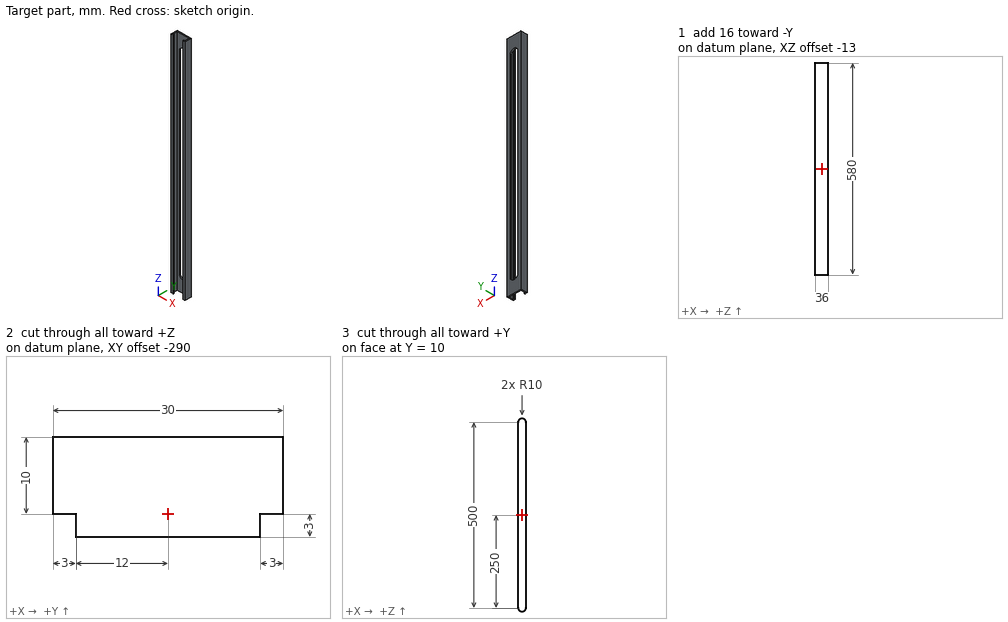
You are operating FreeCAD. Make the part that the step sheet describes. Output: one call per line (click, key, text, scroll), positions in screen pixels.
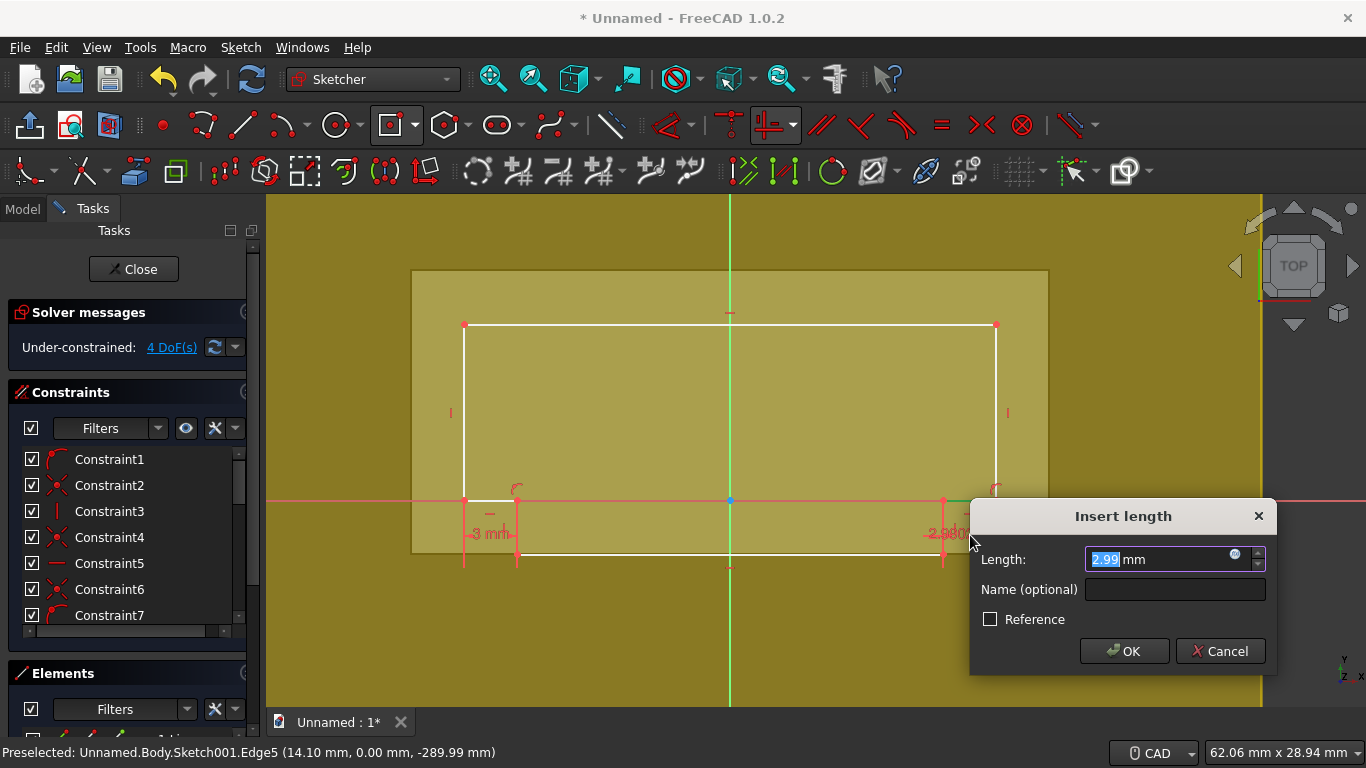
text(3)
key(Return)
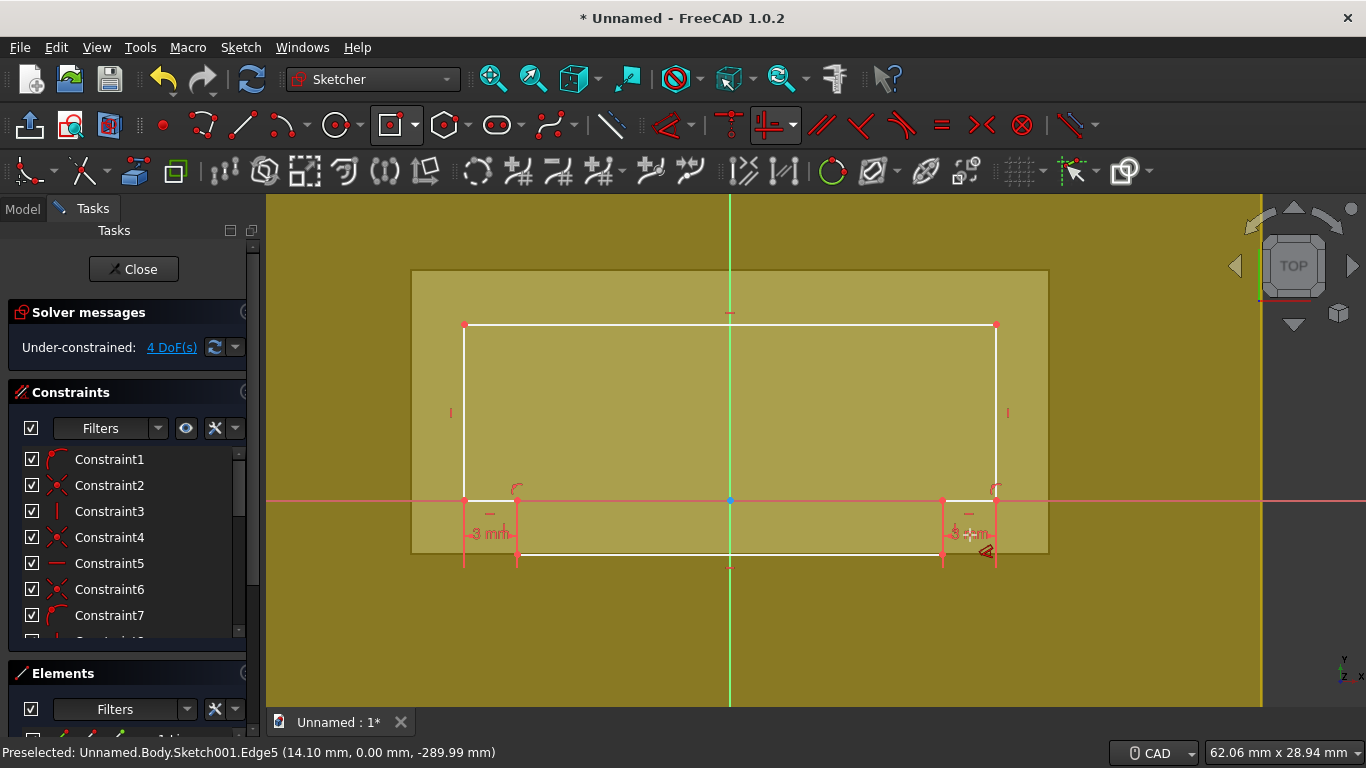
click(943, 517)
click(885, 528)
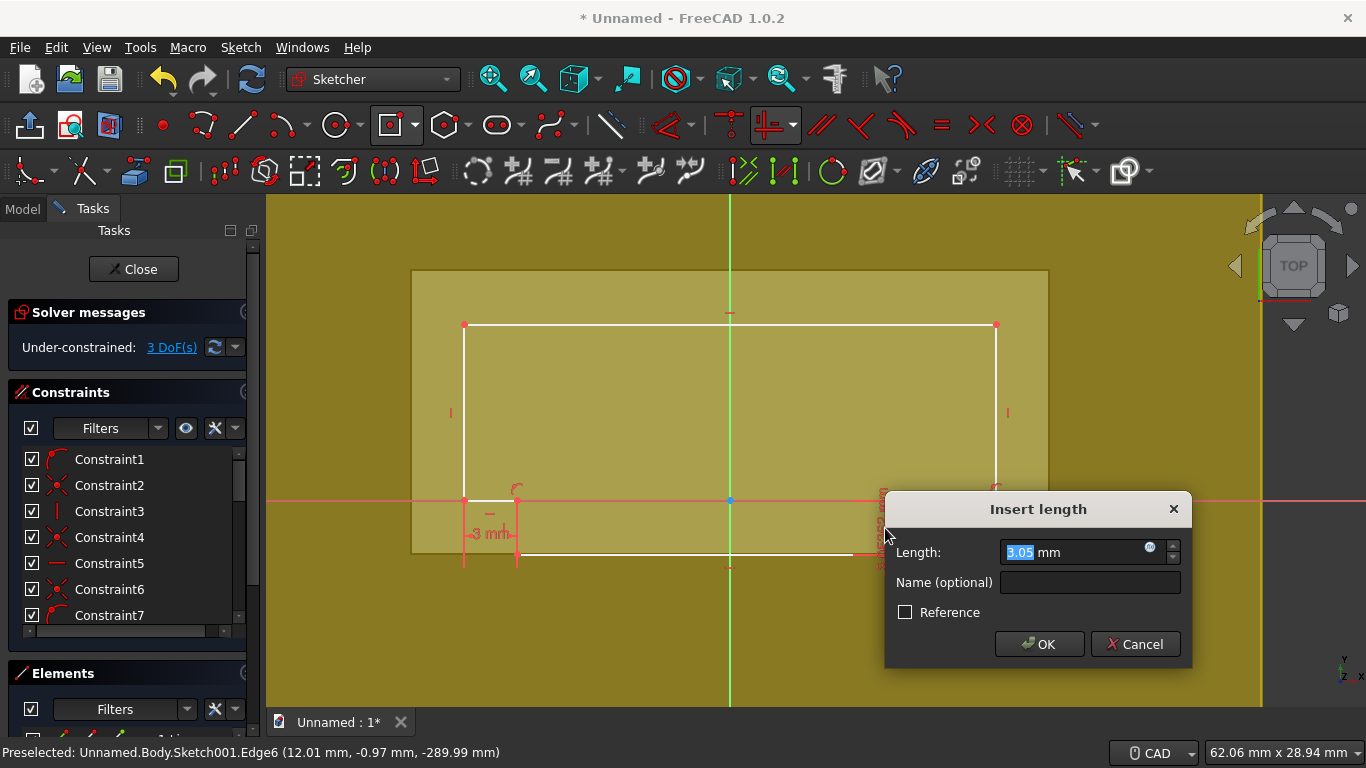
text(3)
key(Return)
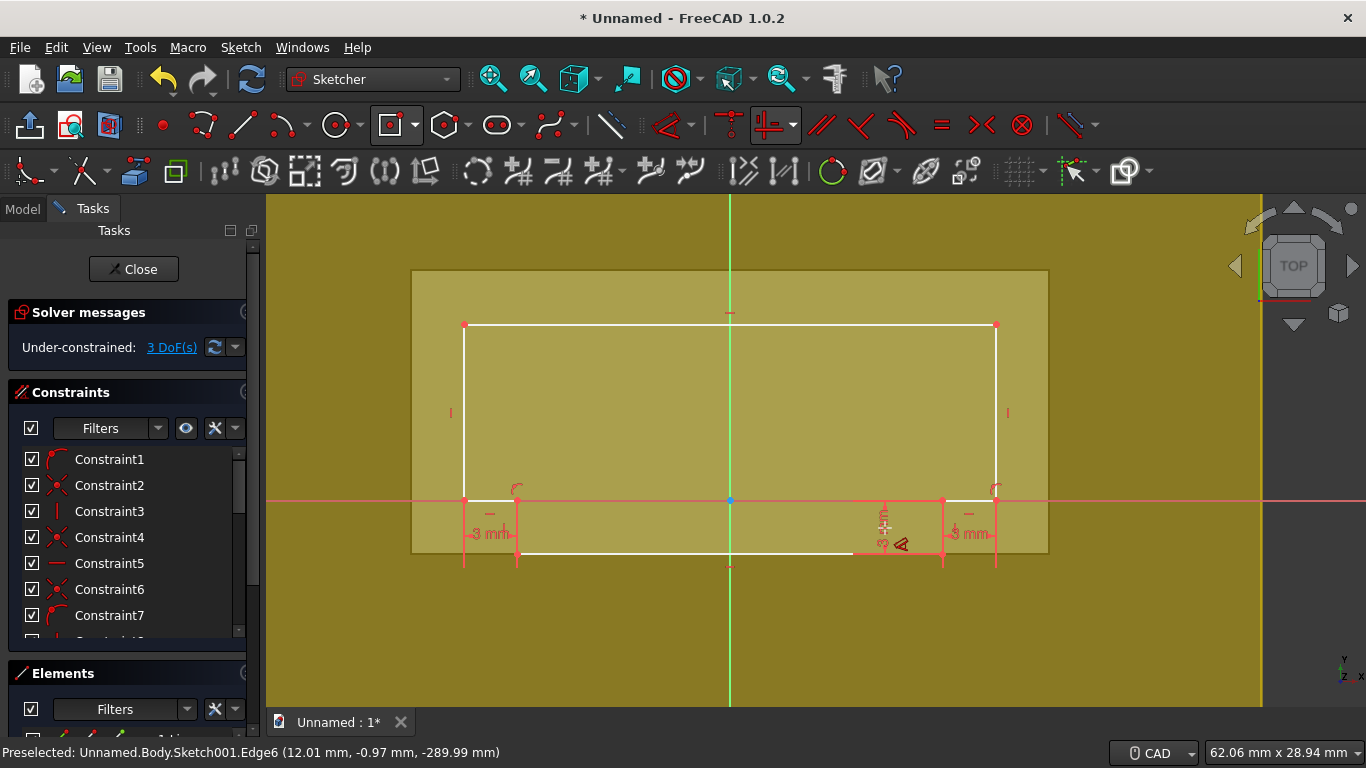
click(464, 448)
click(430, 413)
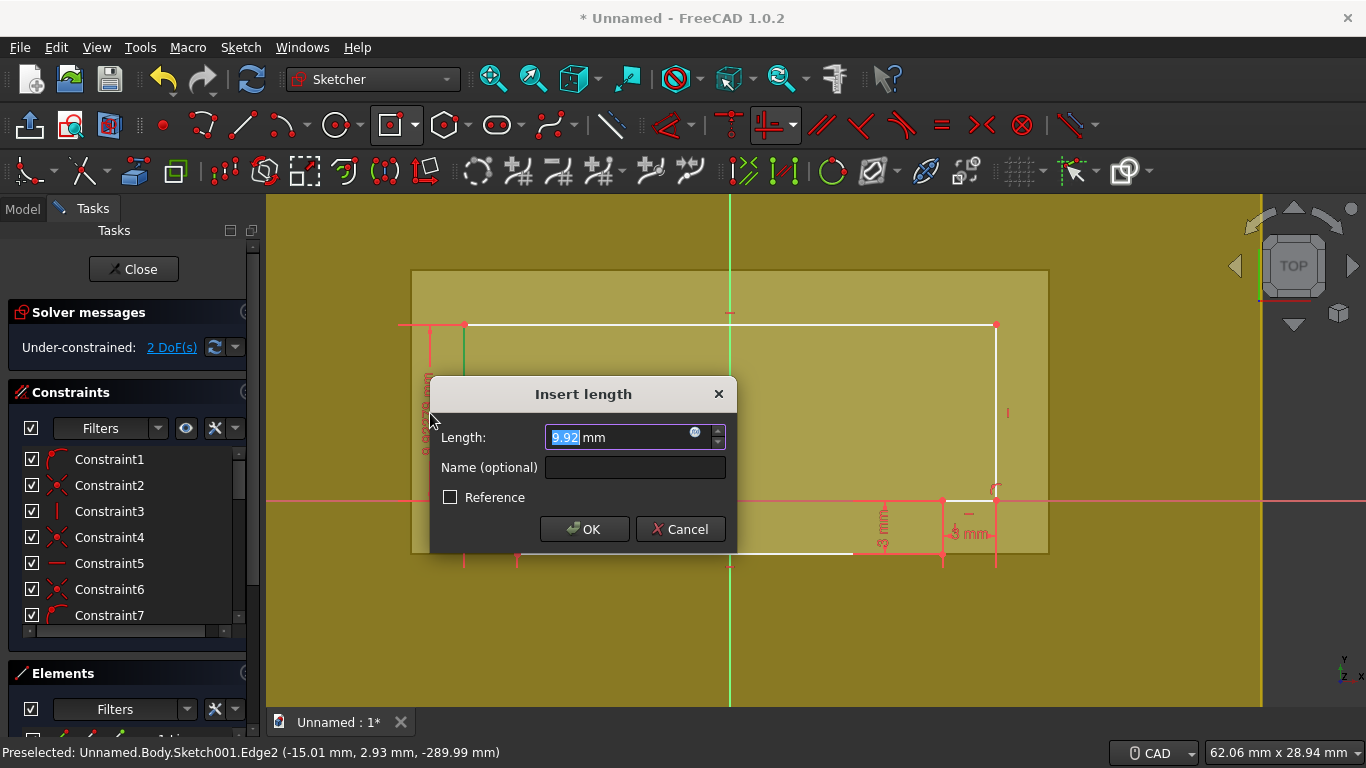
text(10)
key(Return)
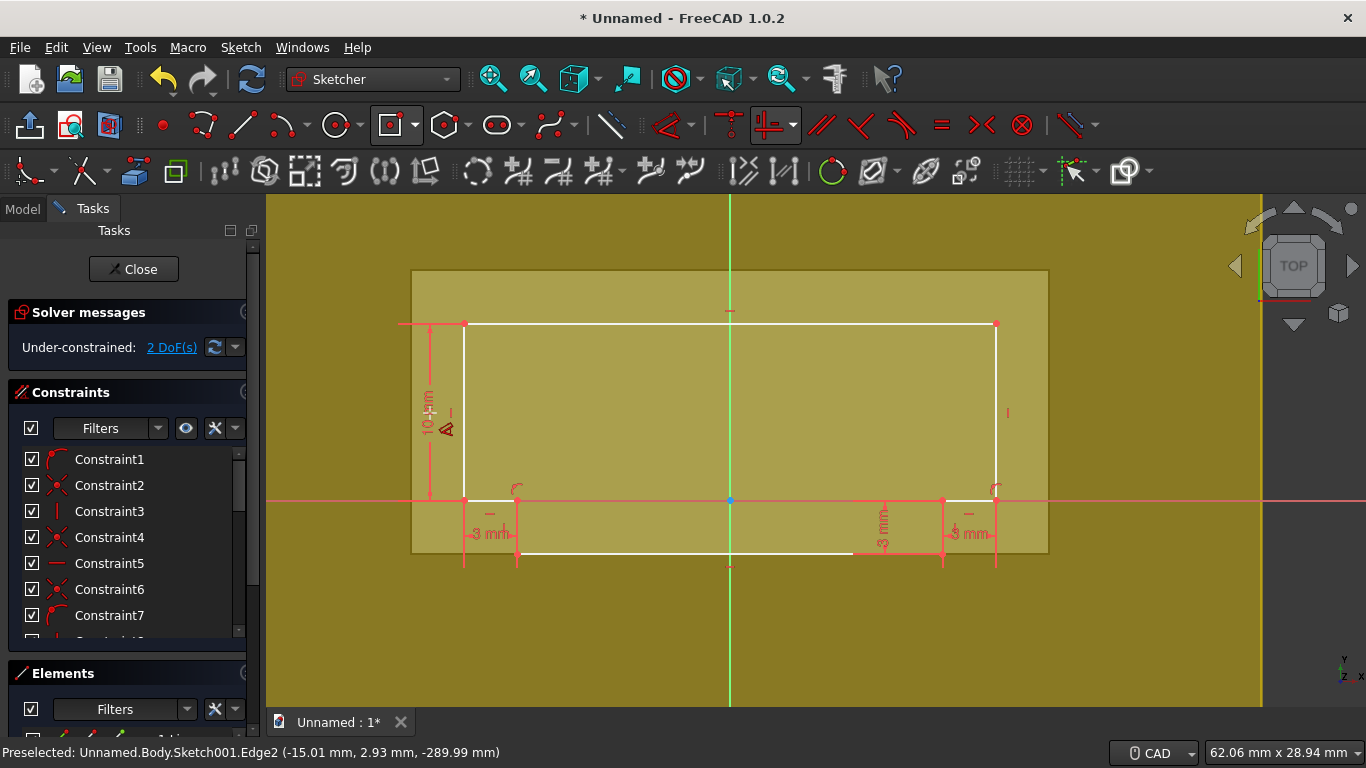
click(624, 324)
click(608, 290)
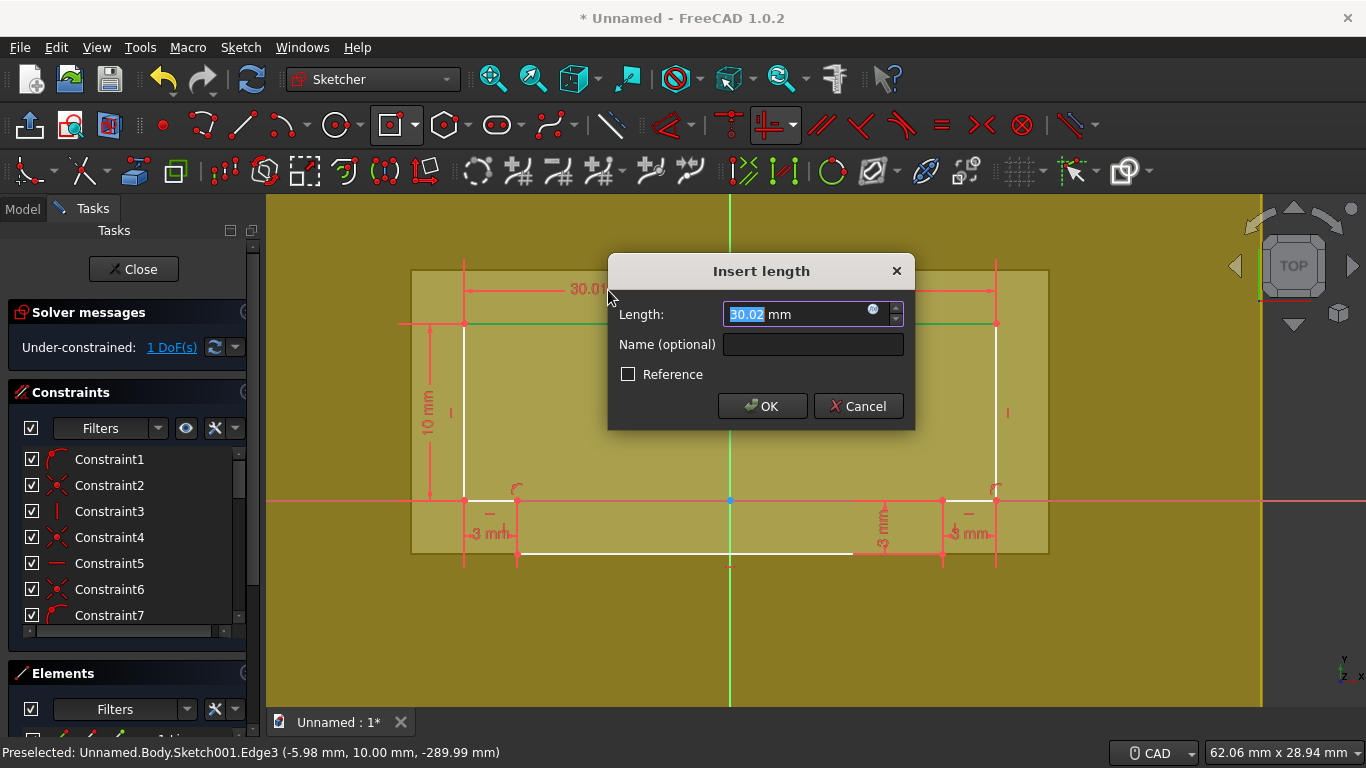
text(30)
key(Return)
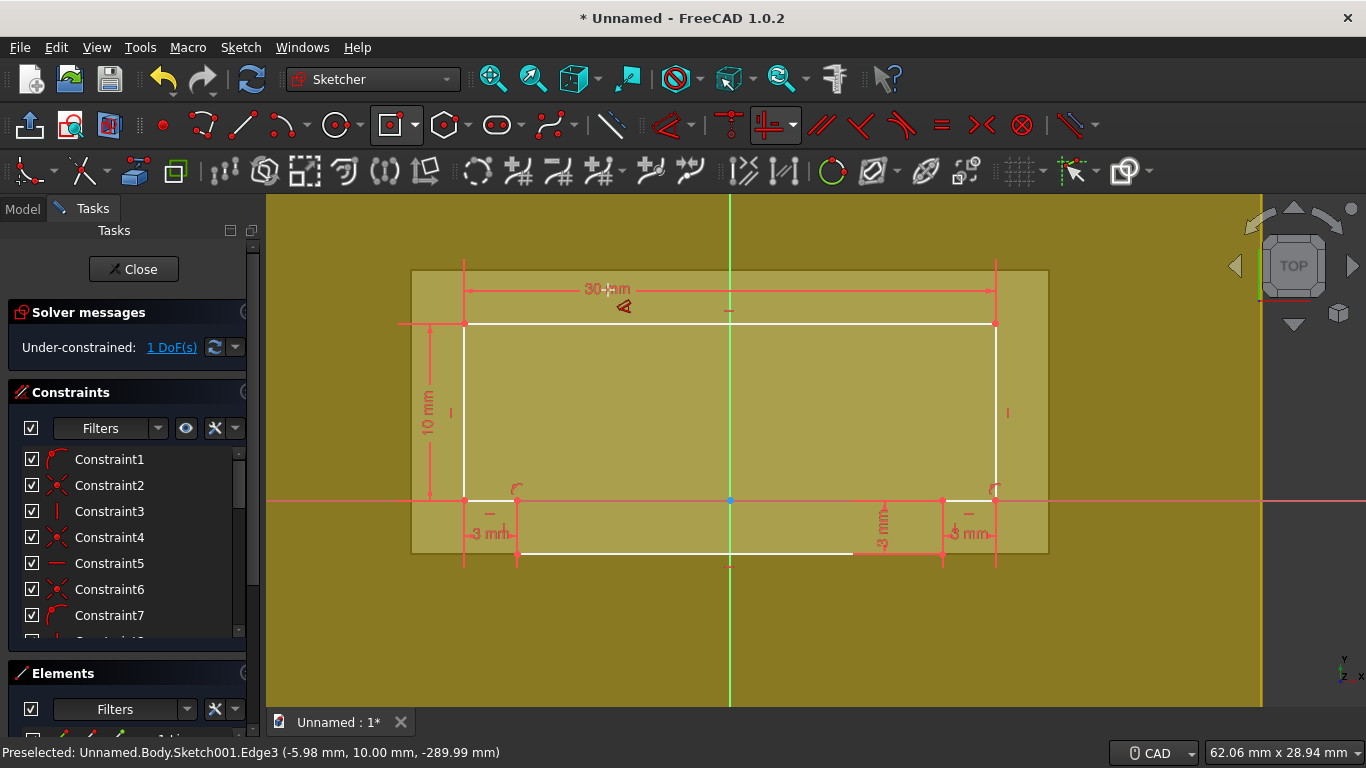
click(517, 501)
click(624, 535)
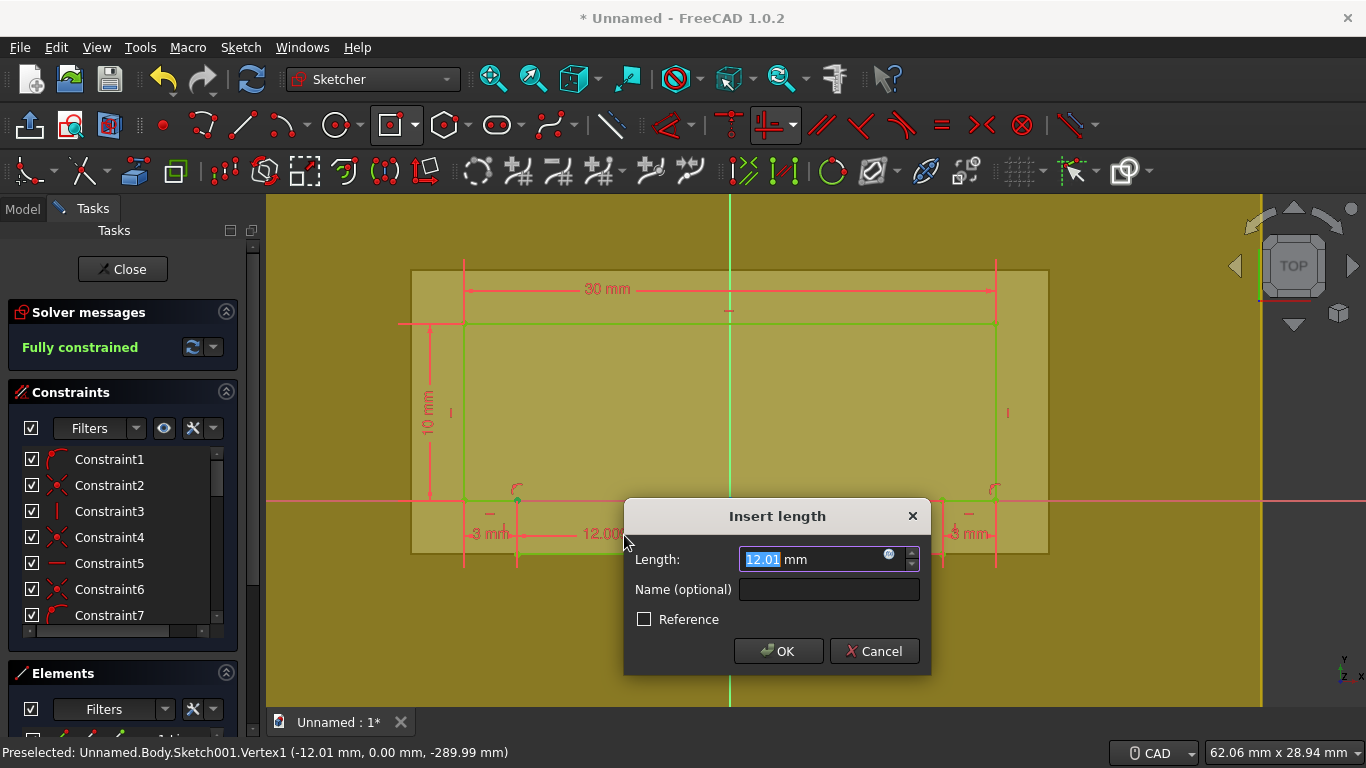
text(12)
key(Return)
key(Escape)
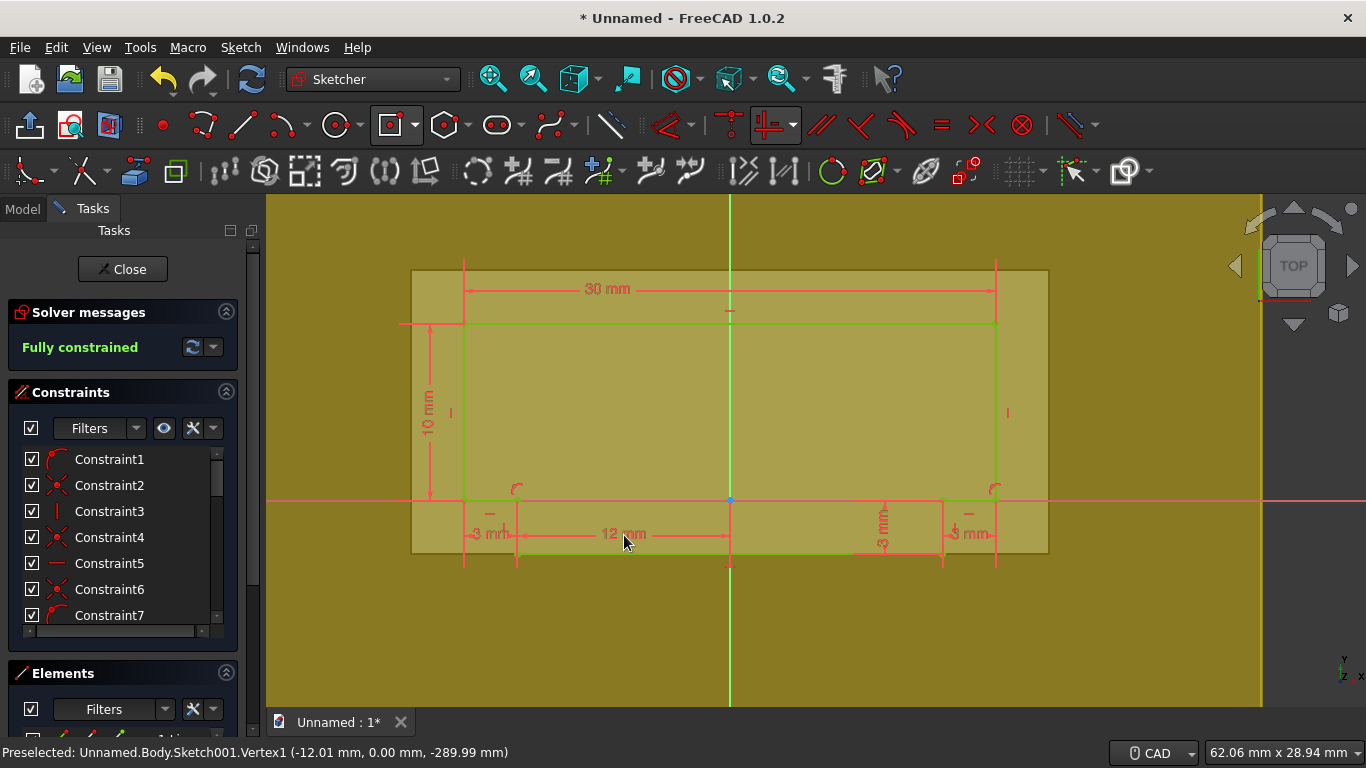
click(123, 269)